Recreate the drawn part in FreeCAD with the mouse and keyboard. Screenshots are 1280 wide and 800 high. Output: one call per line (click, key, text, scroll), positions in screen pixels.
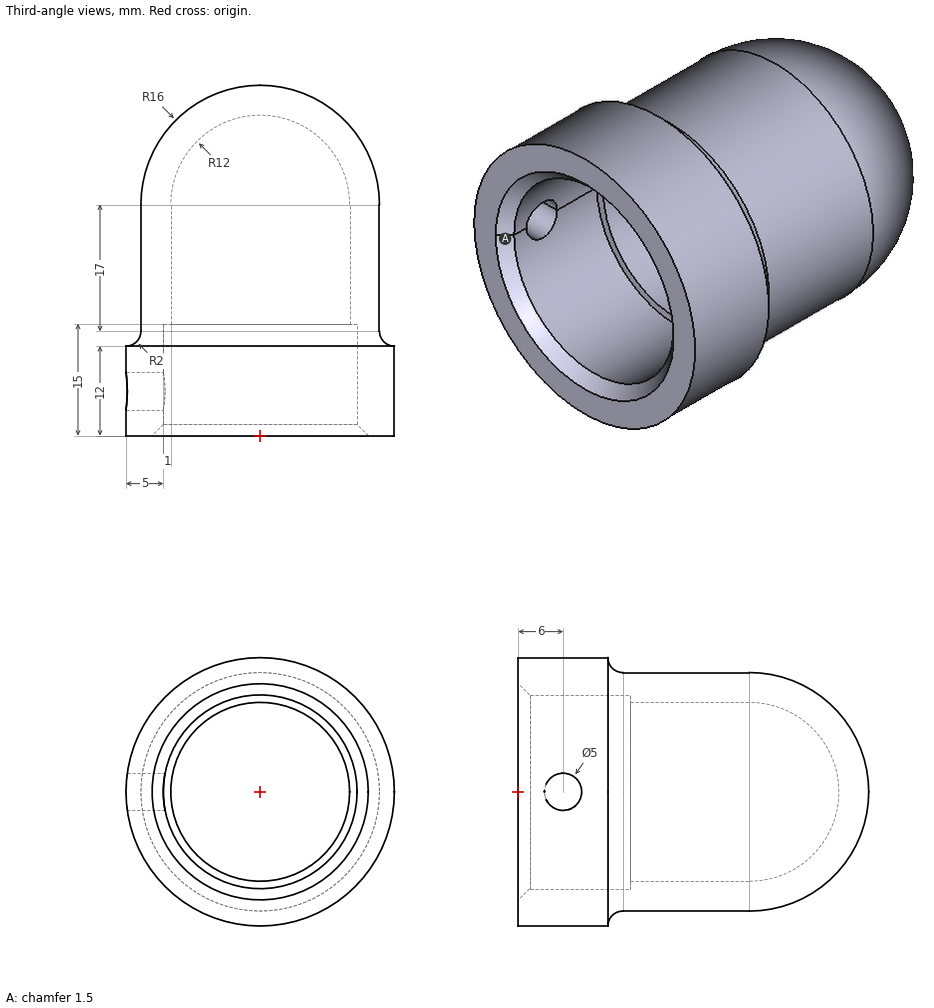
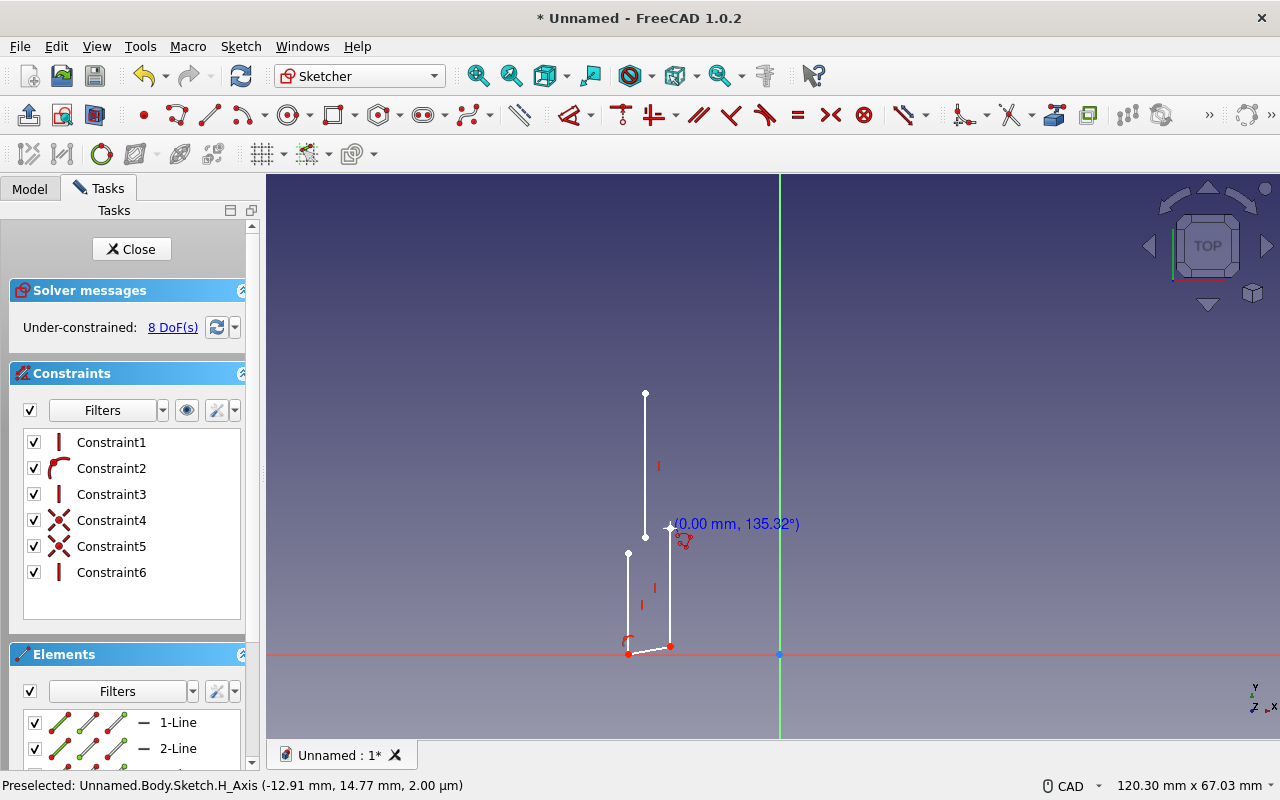
scroll(679, 528, up, 4)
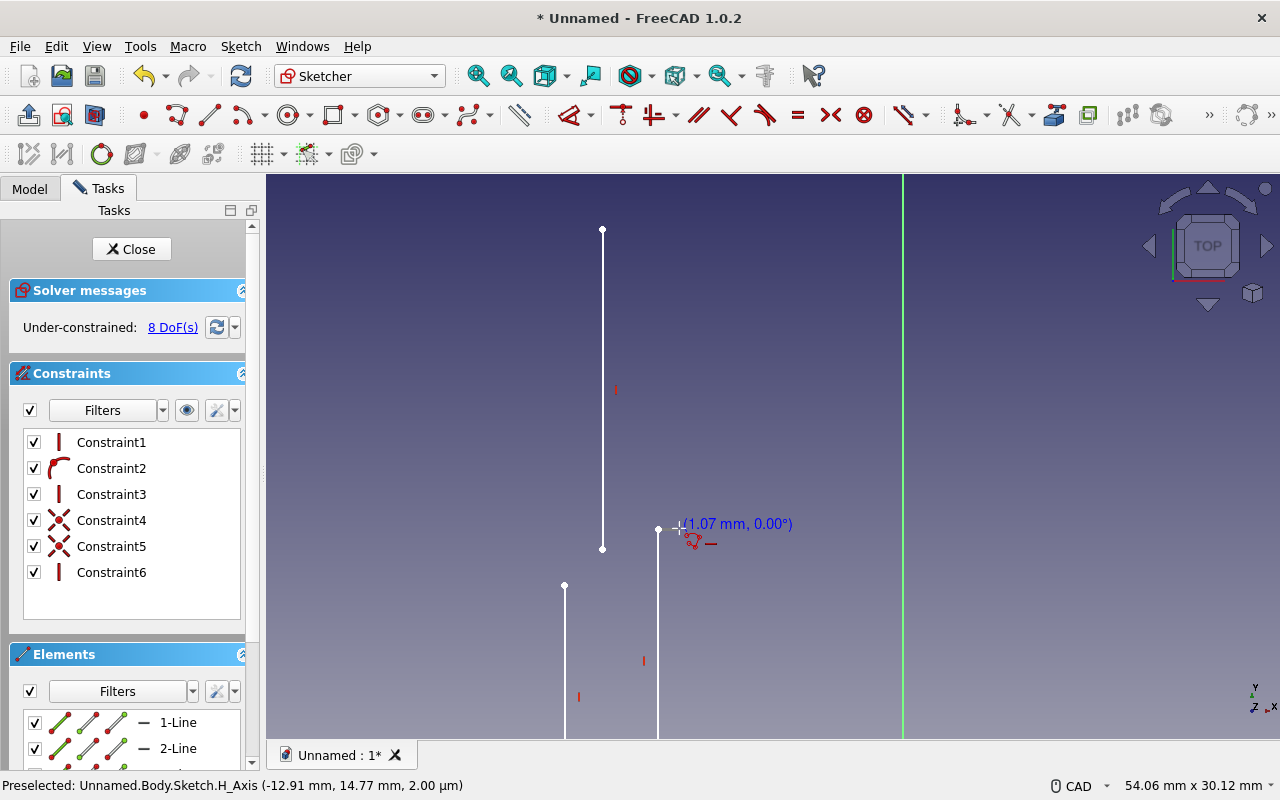
click(678, 527)
click(678, 227)
right_click(678, 227)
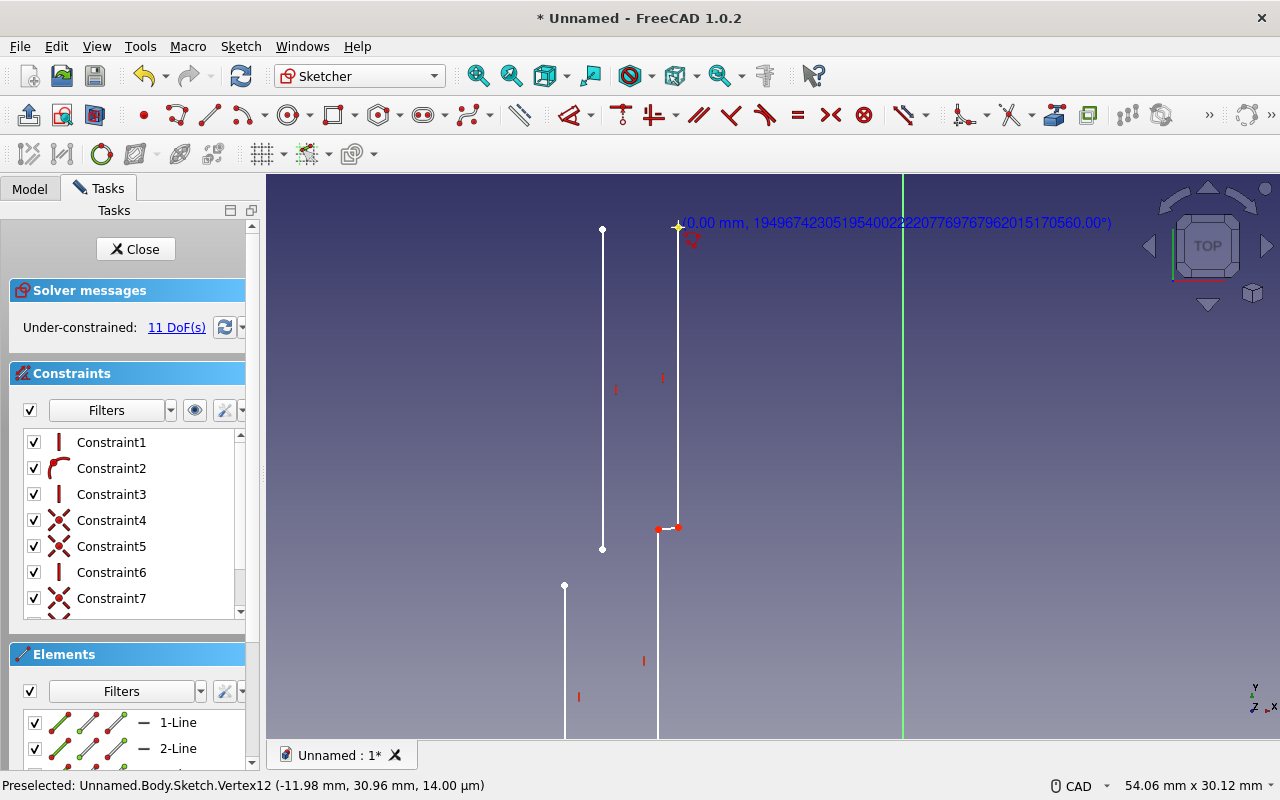
click(210, 116)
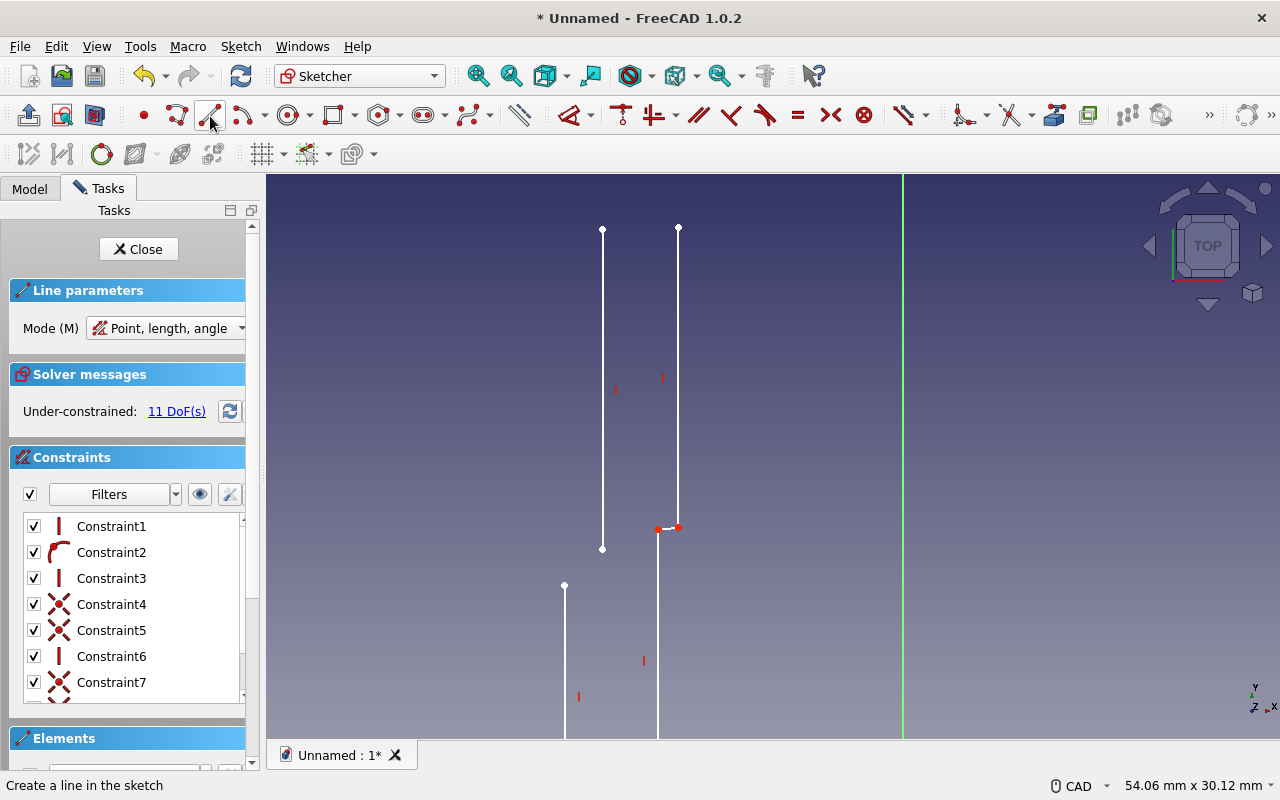
scroll(680, 529, down, 4)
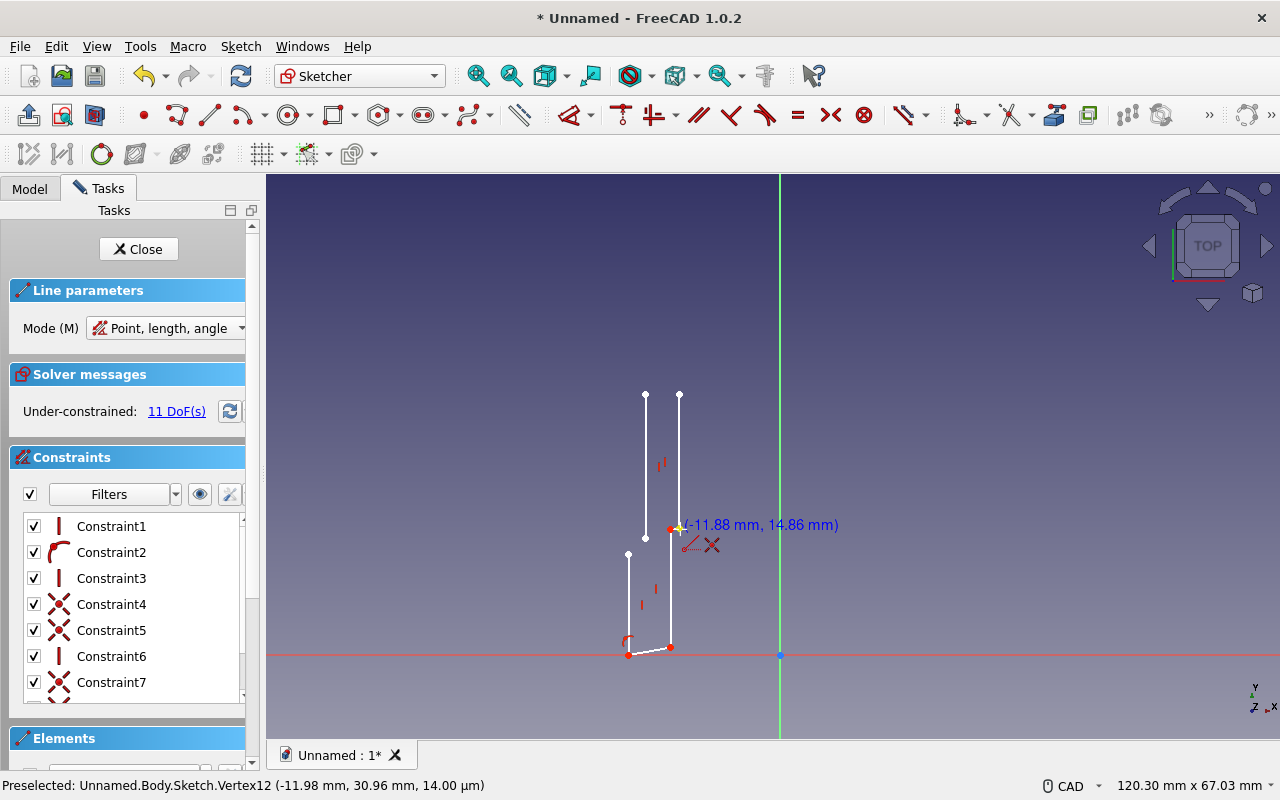
click(780, 293)
click(771, 259)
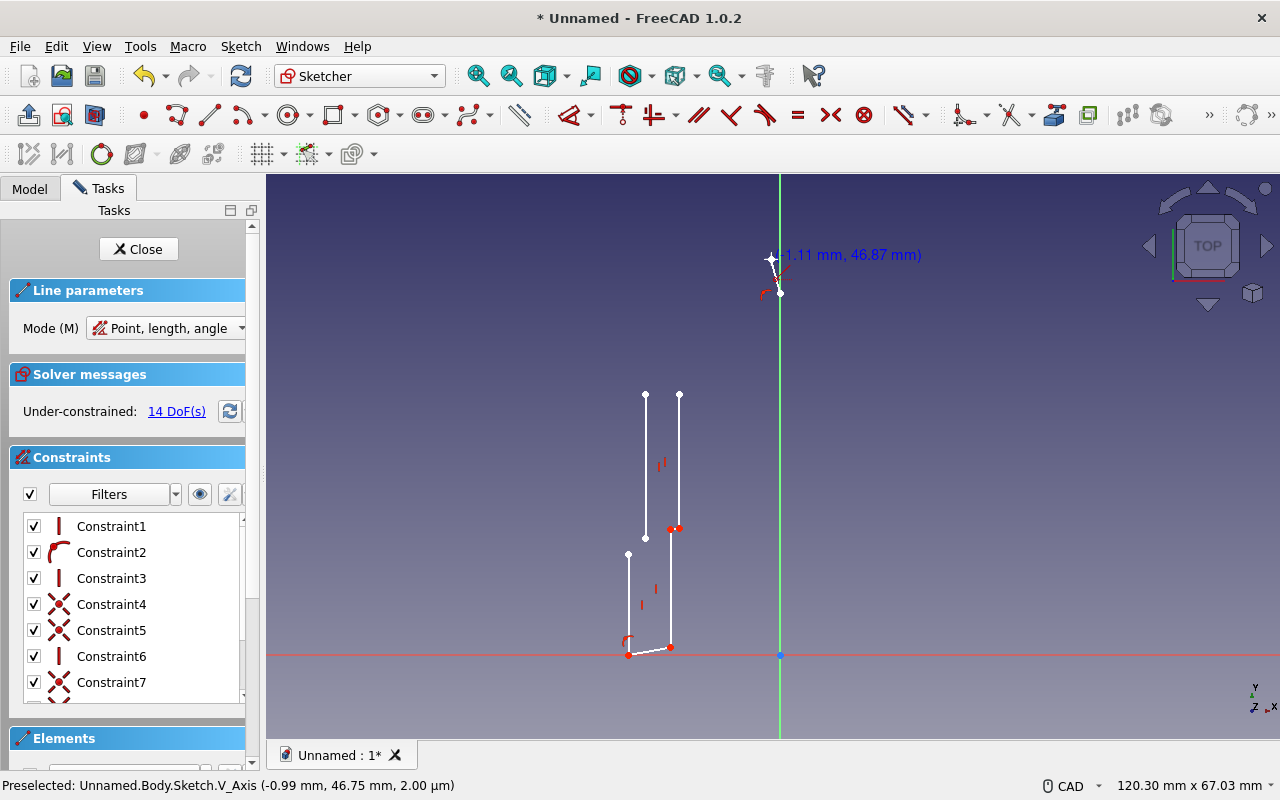
click(264, 116)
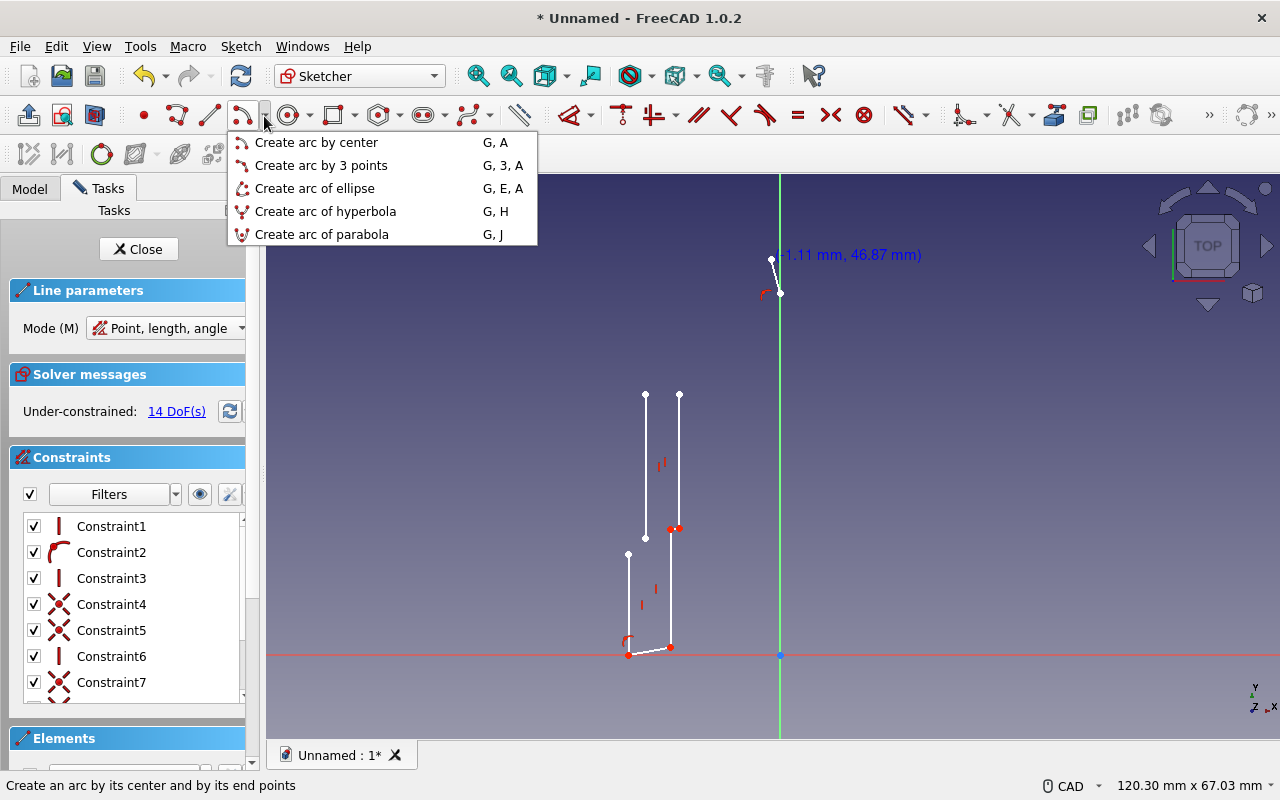
click(382, 166)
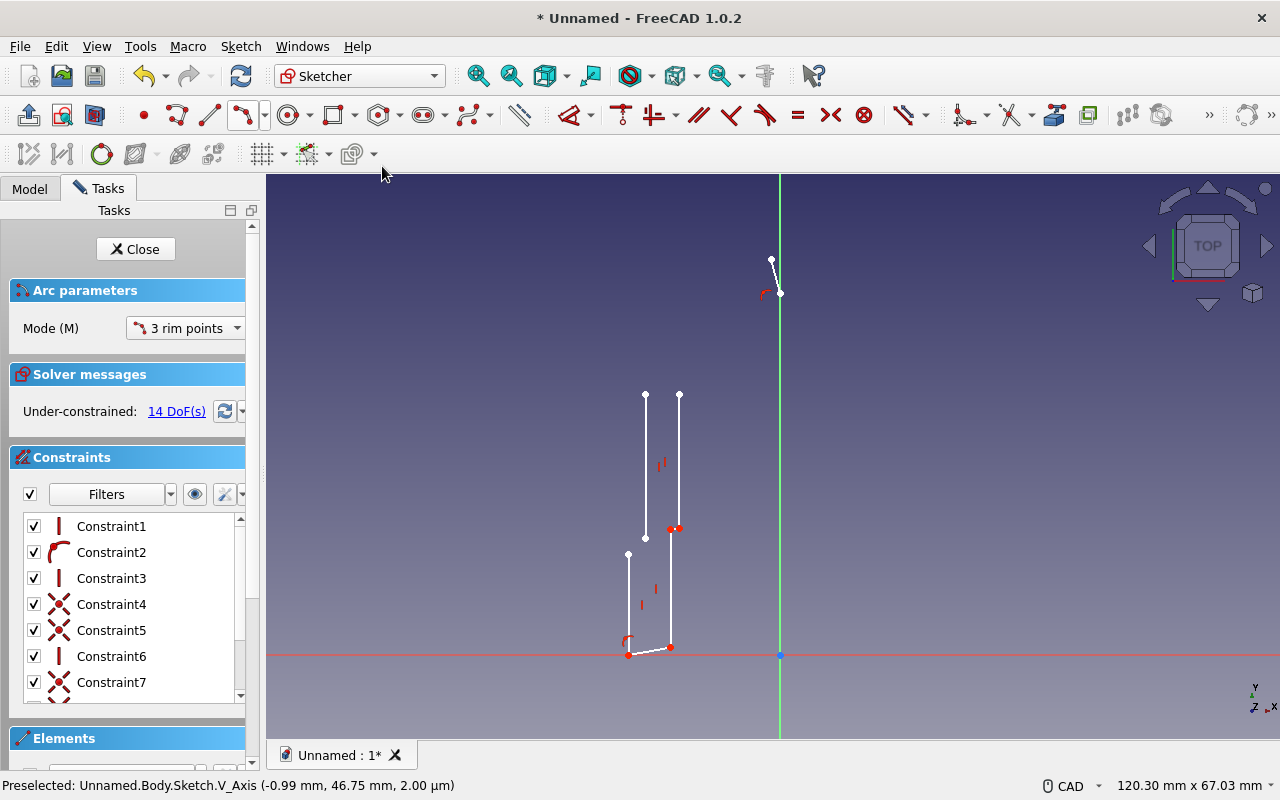
click(646, 539)
click(629, 555)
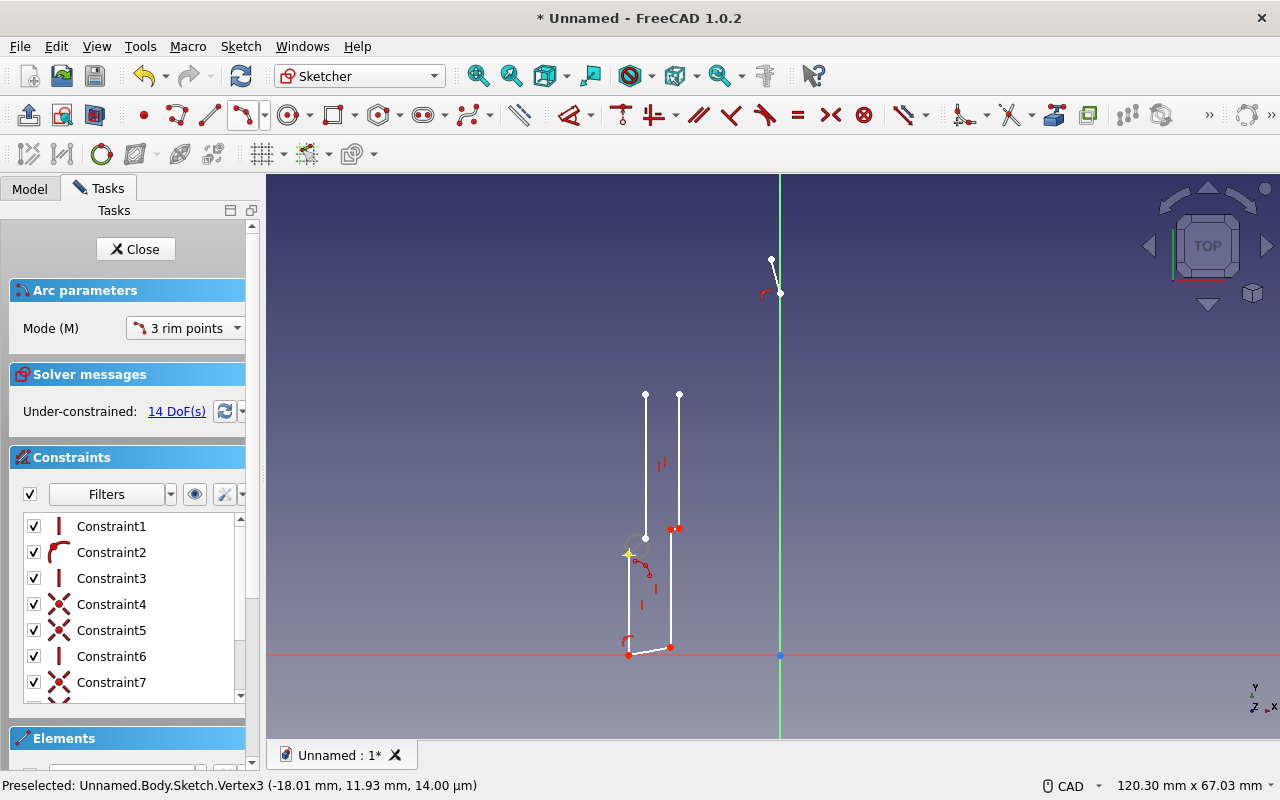
scroll(641, 549, up, 6)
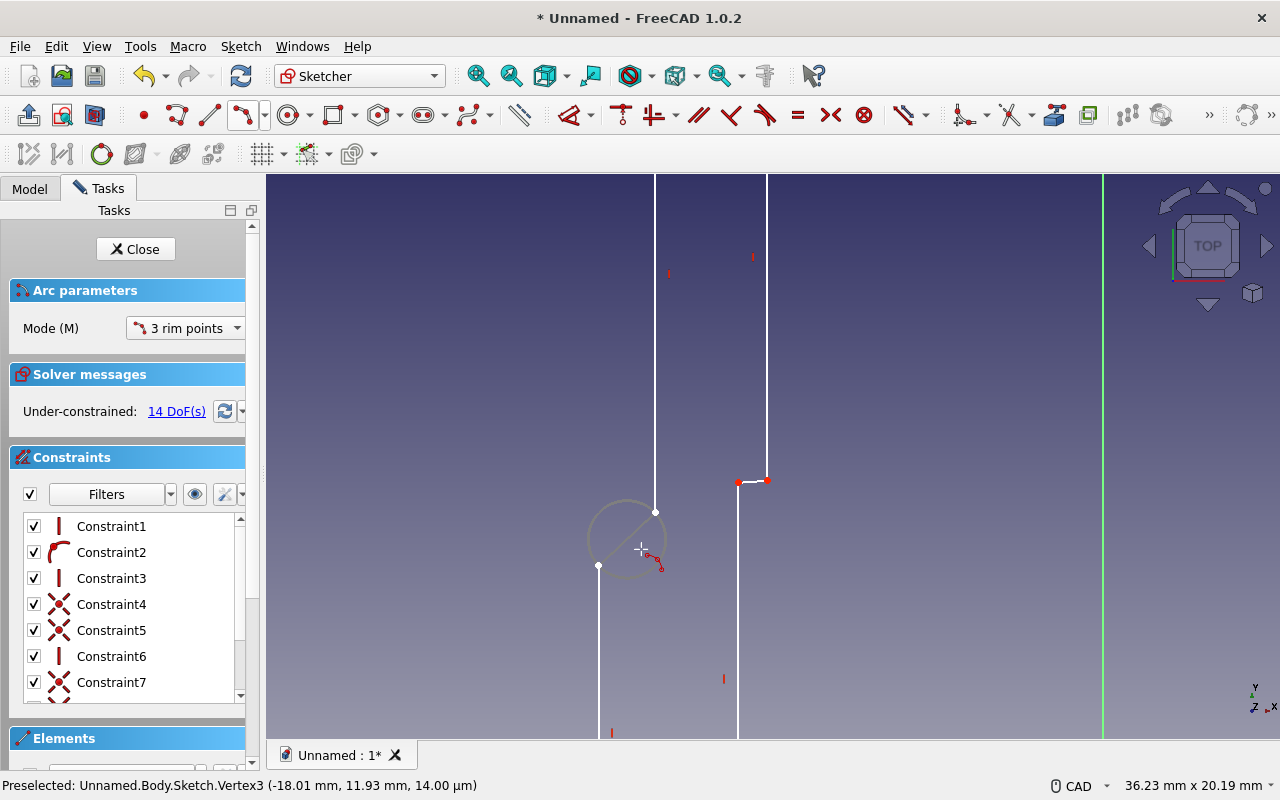
click(639, 547)